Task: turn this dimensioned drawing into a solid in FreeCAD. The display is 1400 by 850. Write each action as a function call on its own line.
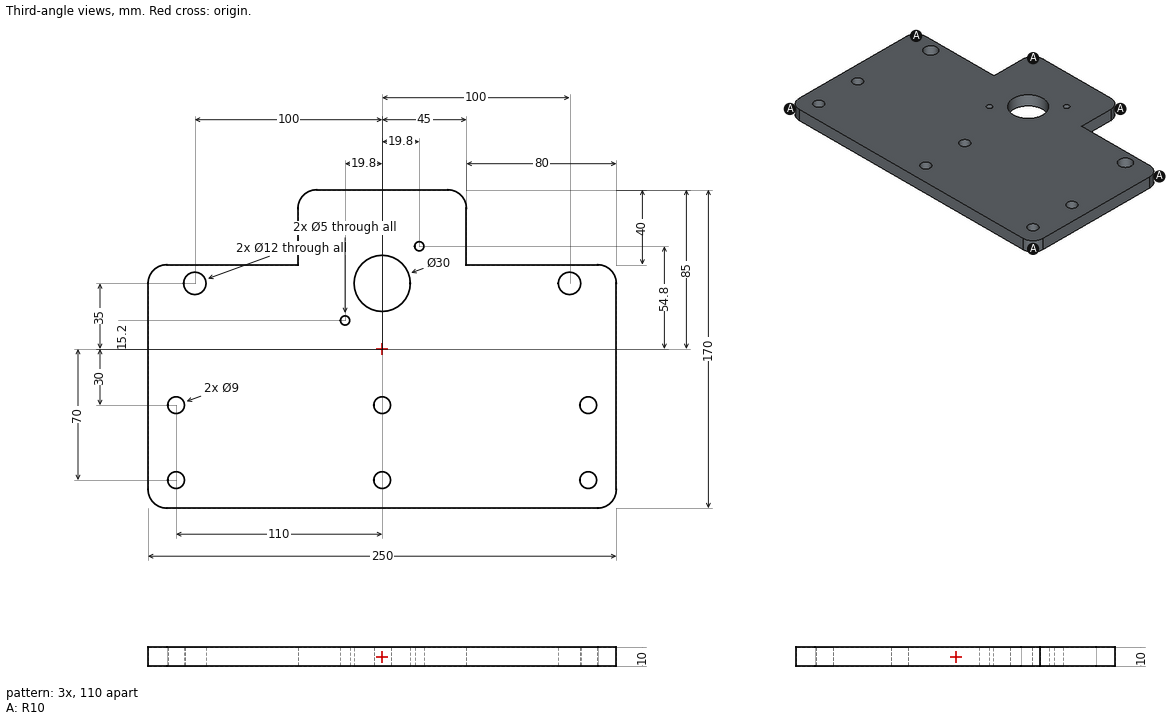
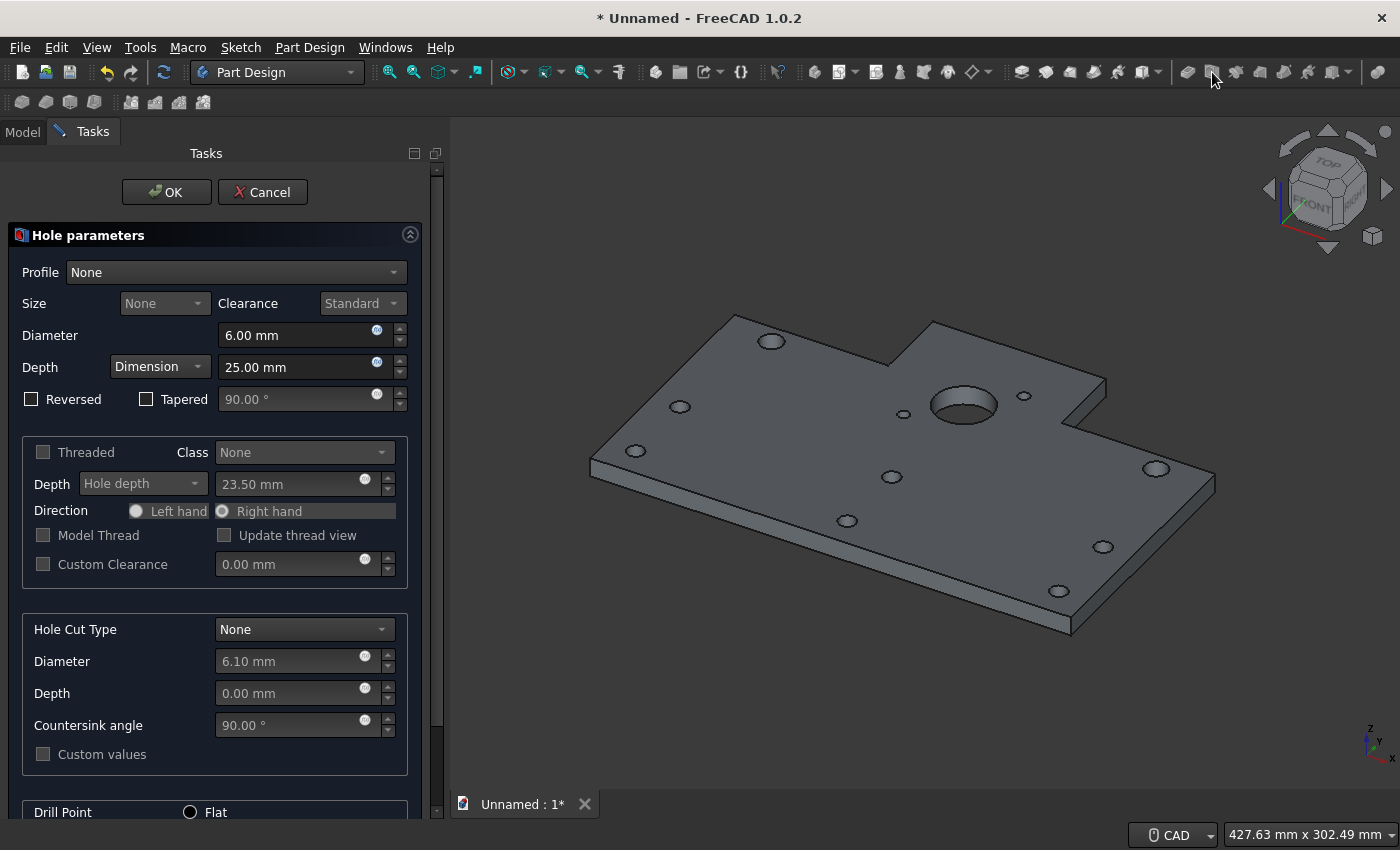
triple_click(305, 335)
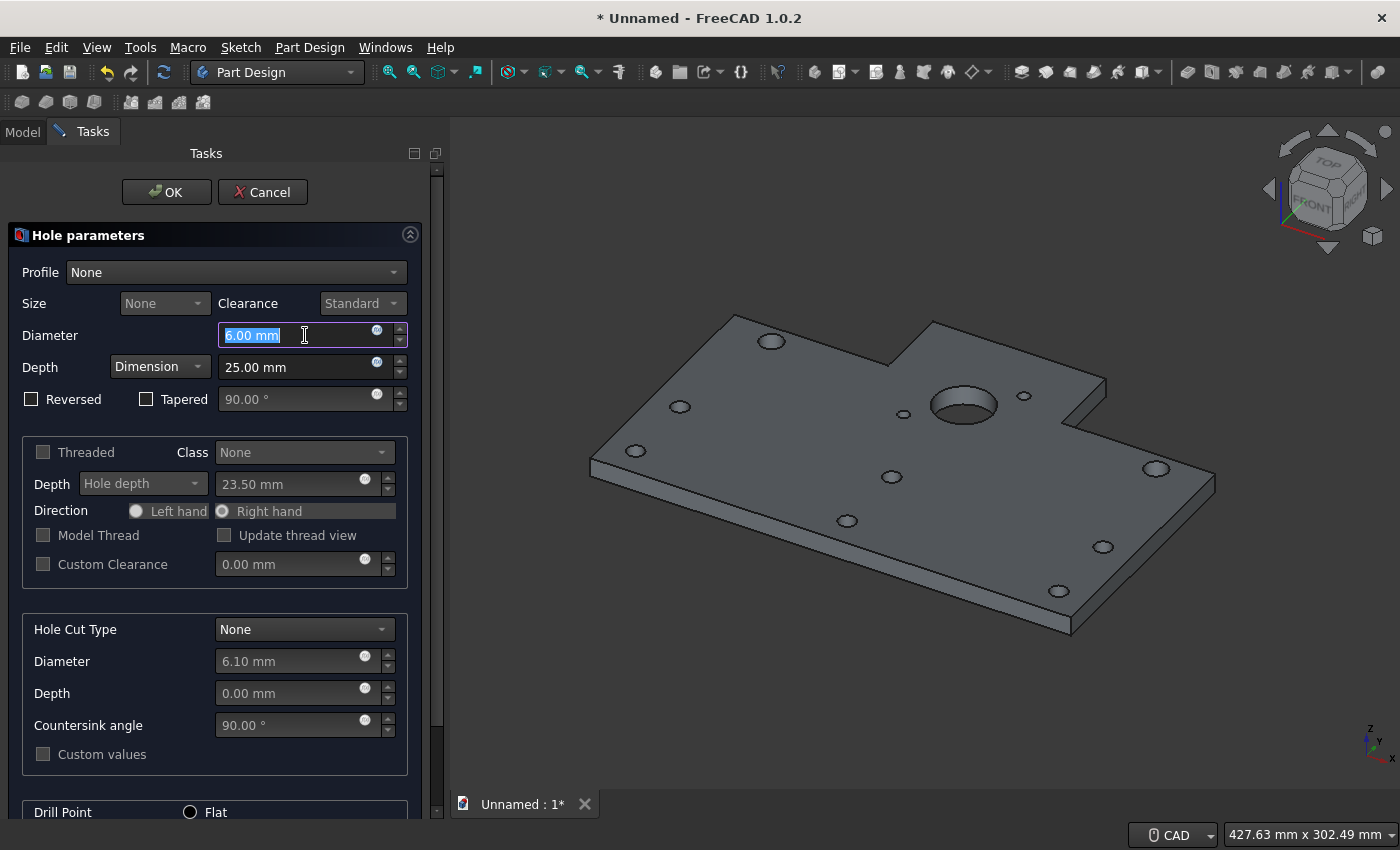
text(5)
key(Tab)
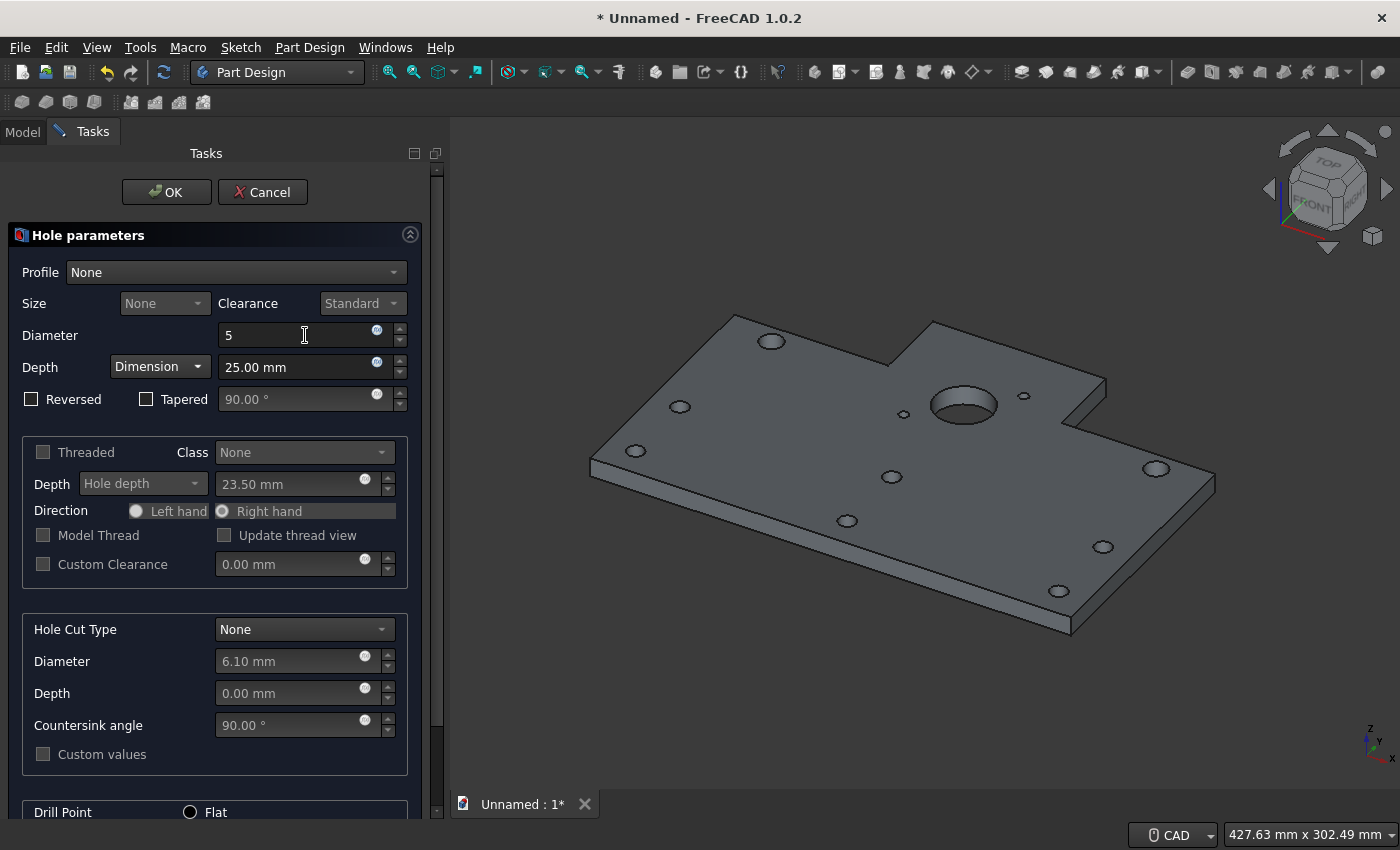
click(161, 366)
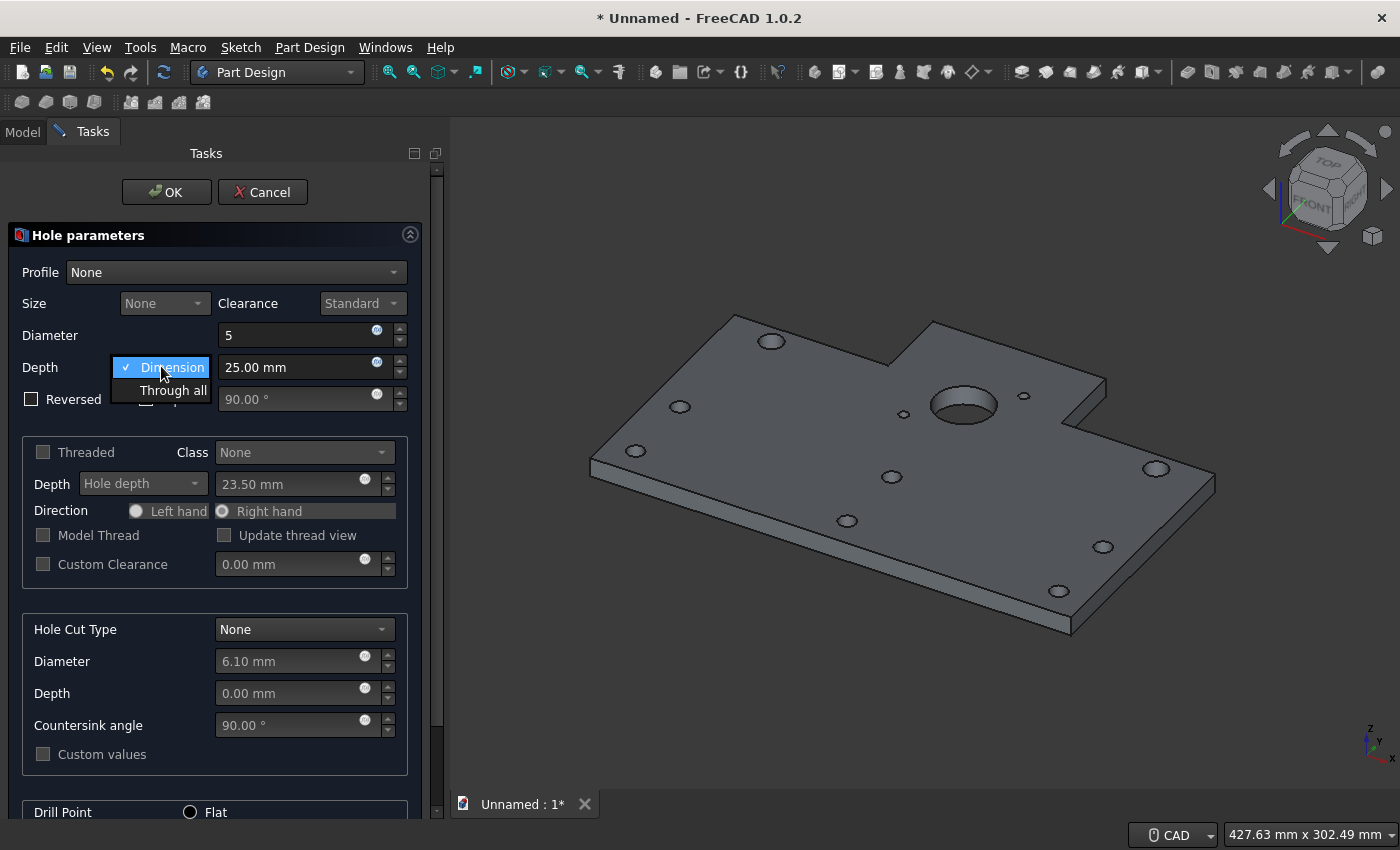
click(160, 390)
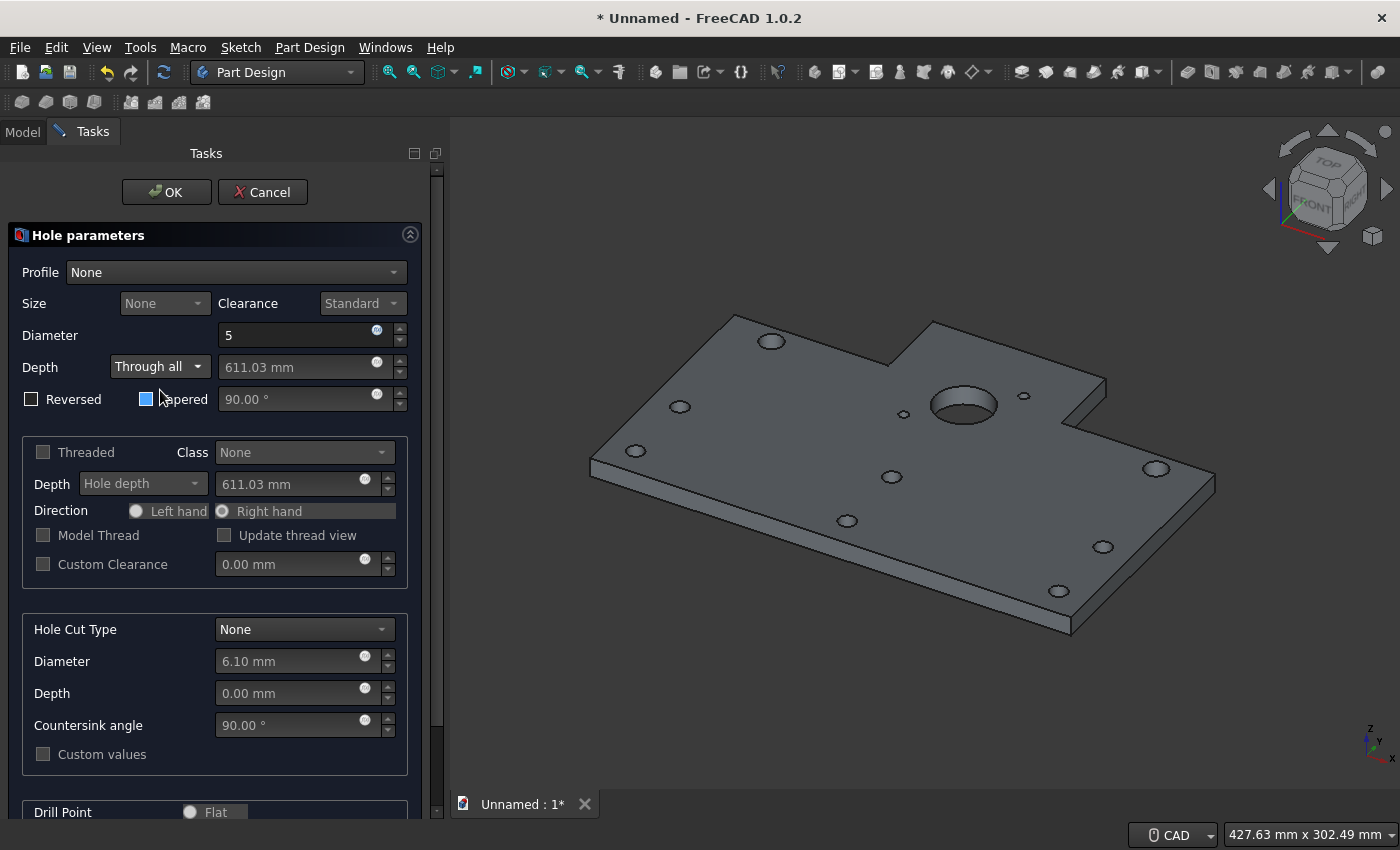
click(167, 192)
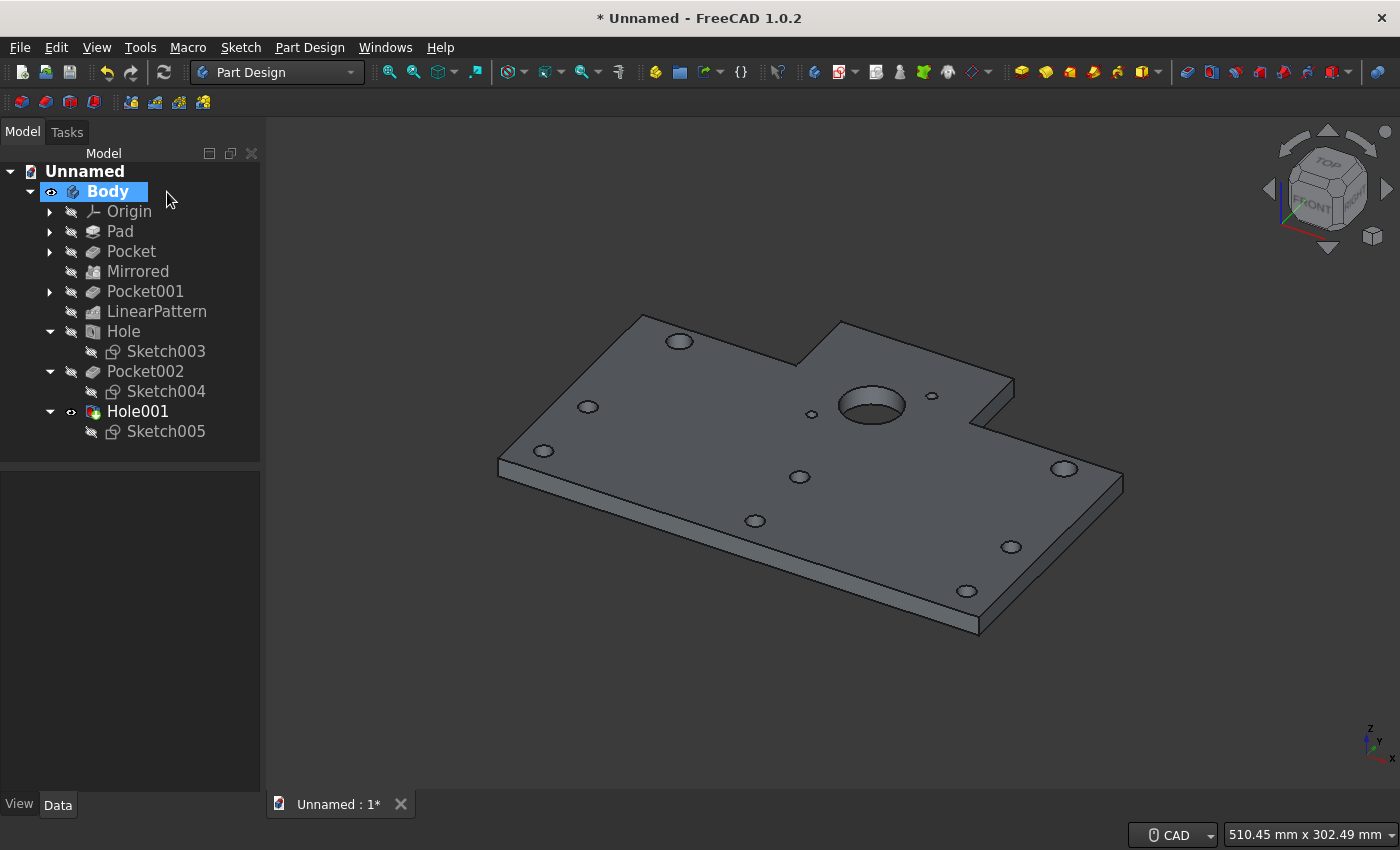
click(979, 625)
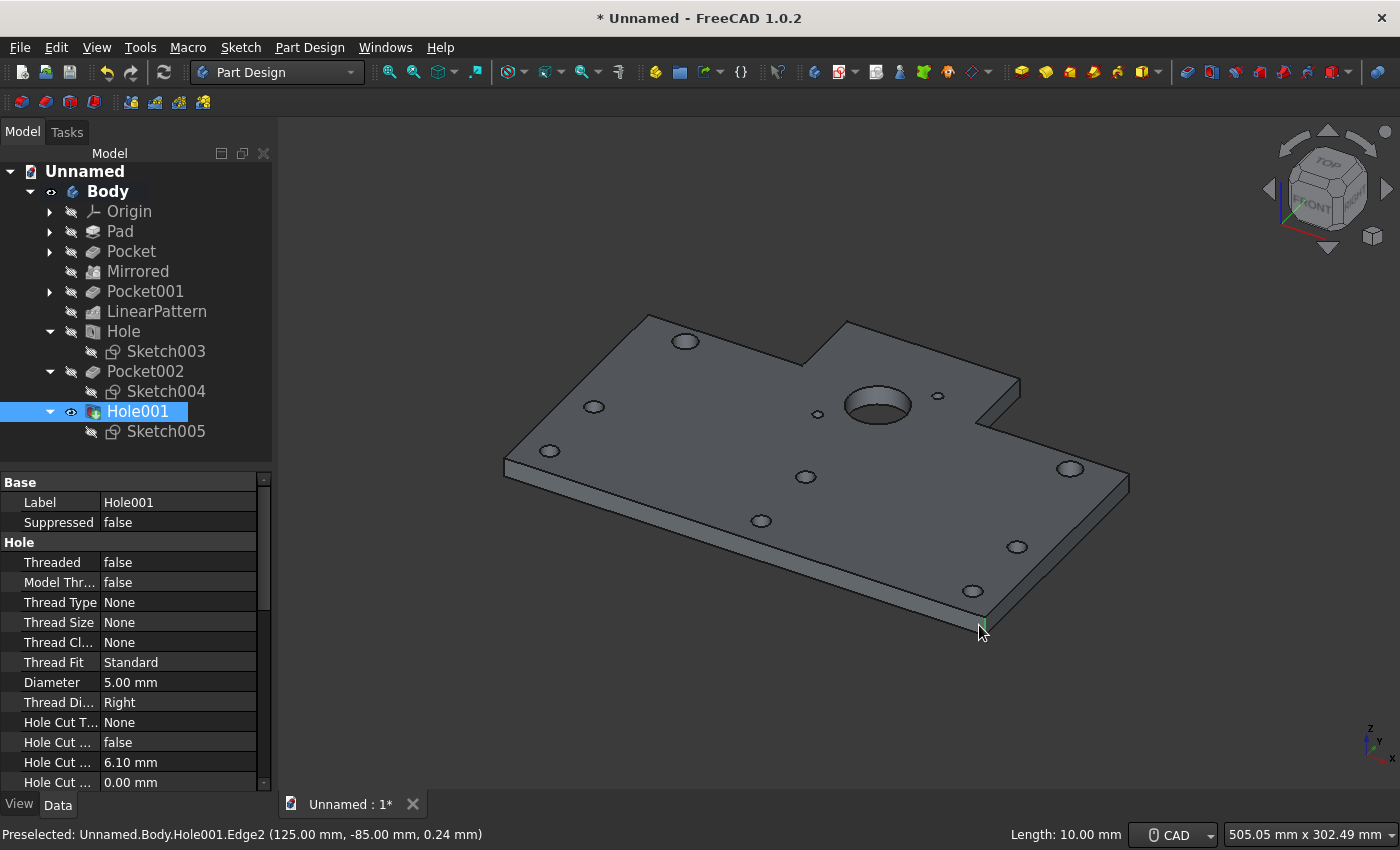
key(0)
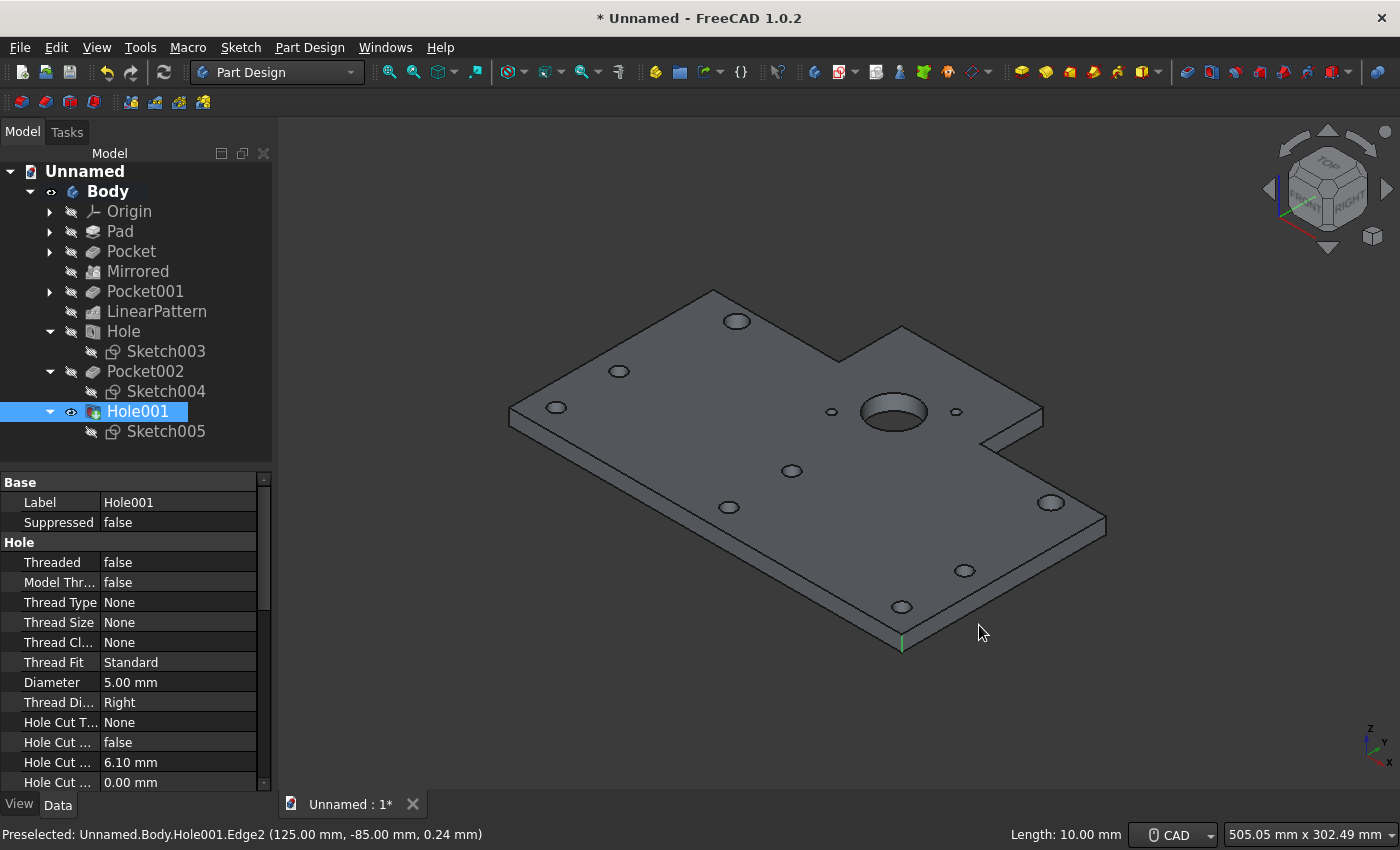
key(2)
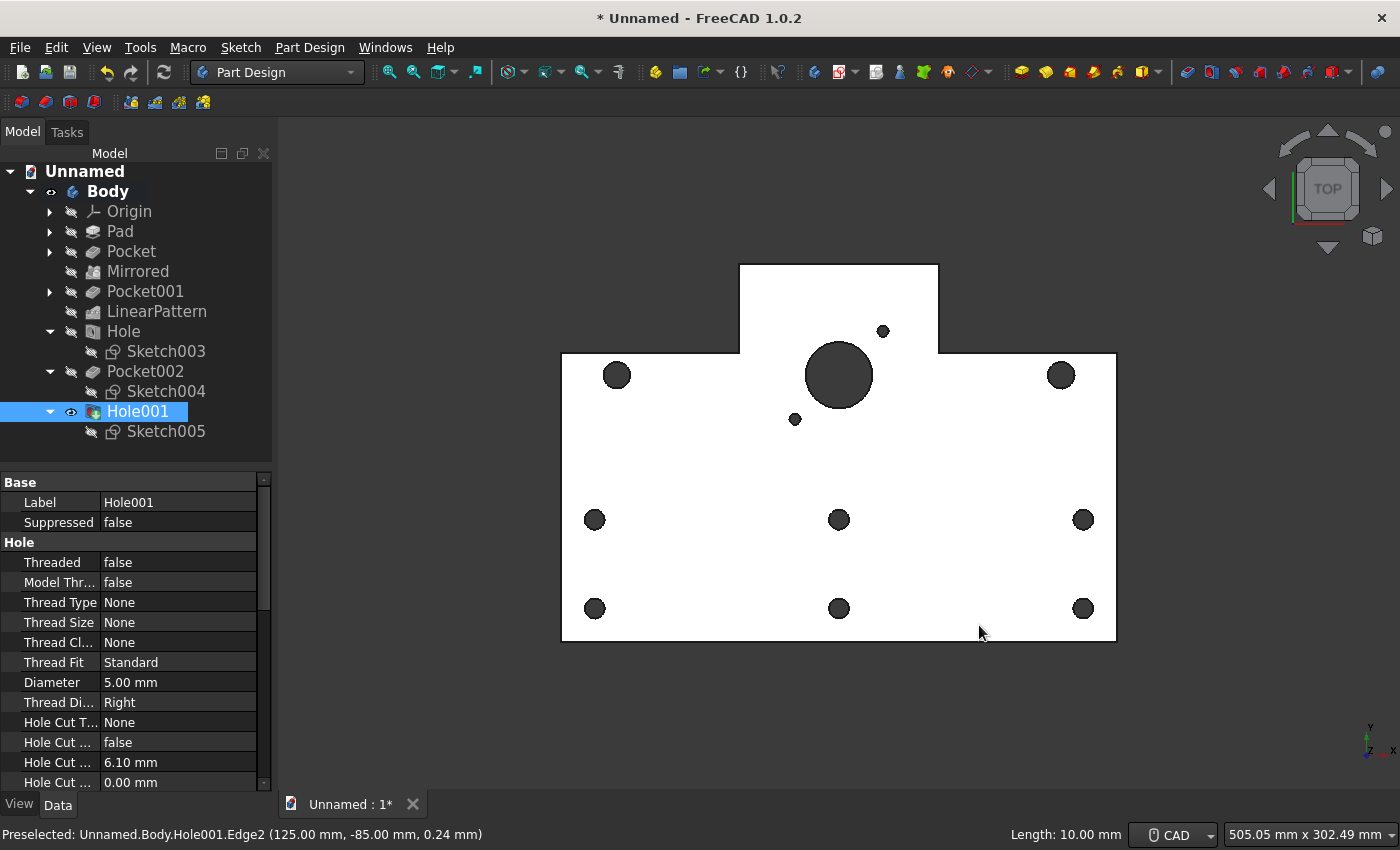
key(1)